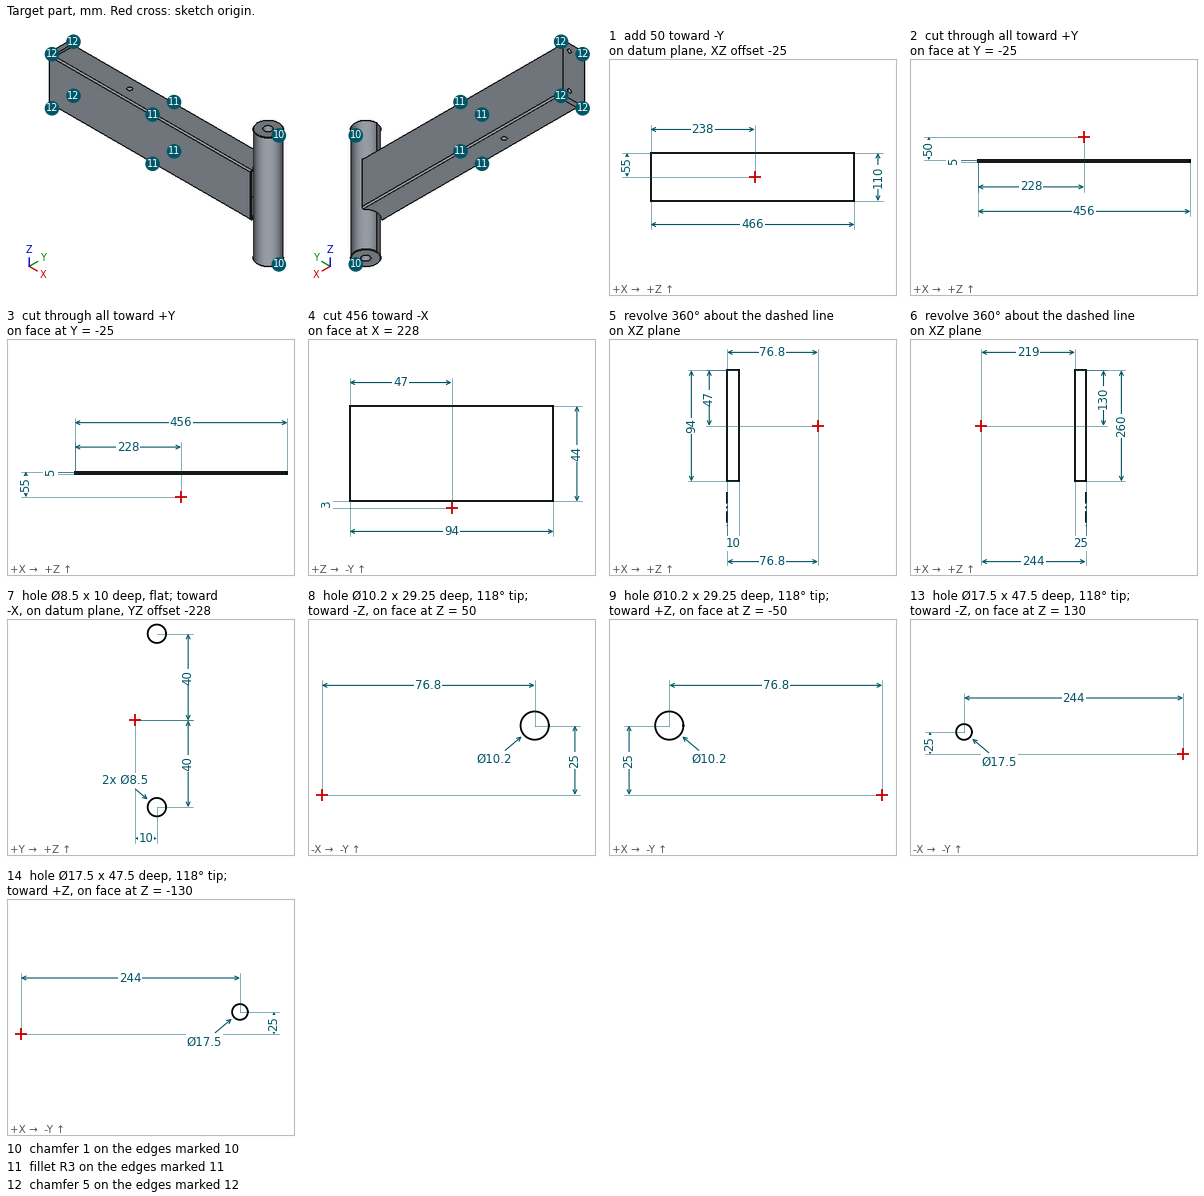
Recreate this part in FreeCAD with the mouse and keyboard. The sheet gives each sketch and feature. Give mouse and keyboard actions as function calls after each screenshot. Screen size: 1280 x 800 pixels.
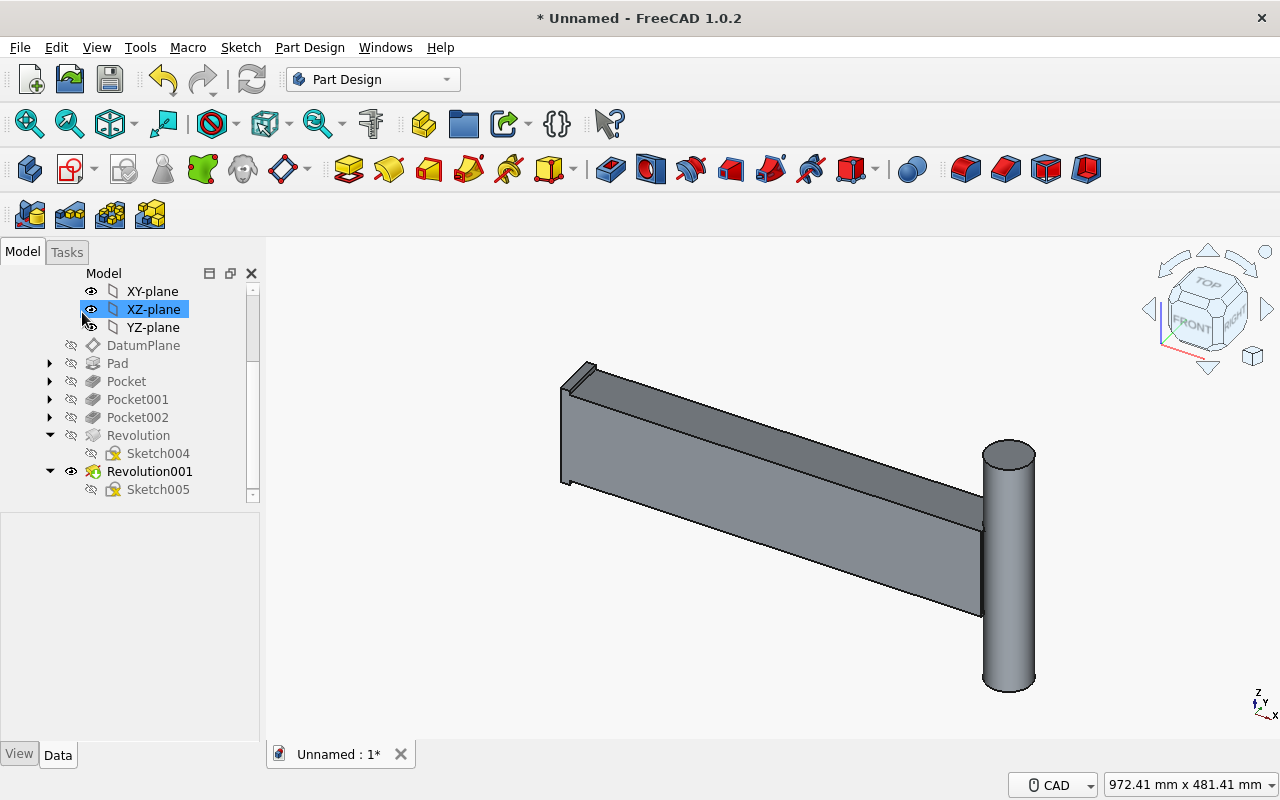
scroll(160, 395, down, 3)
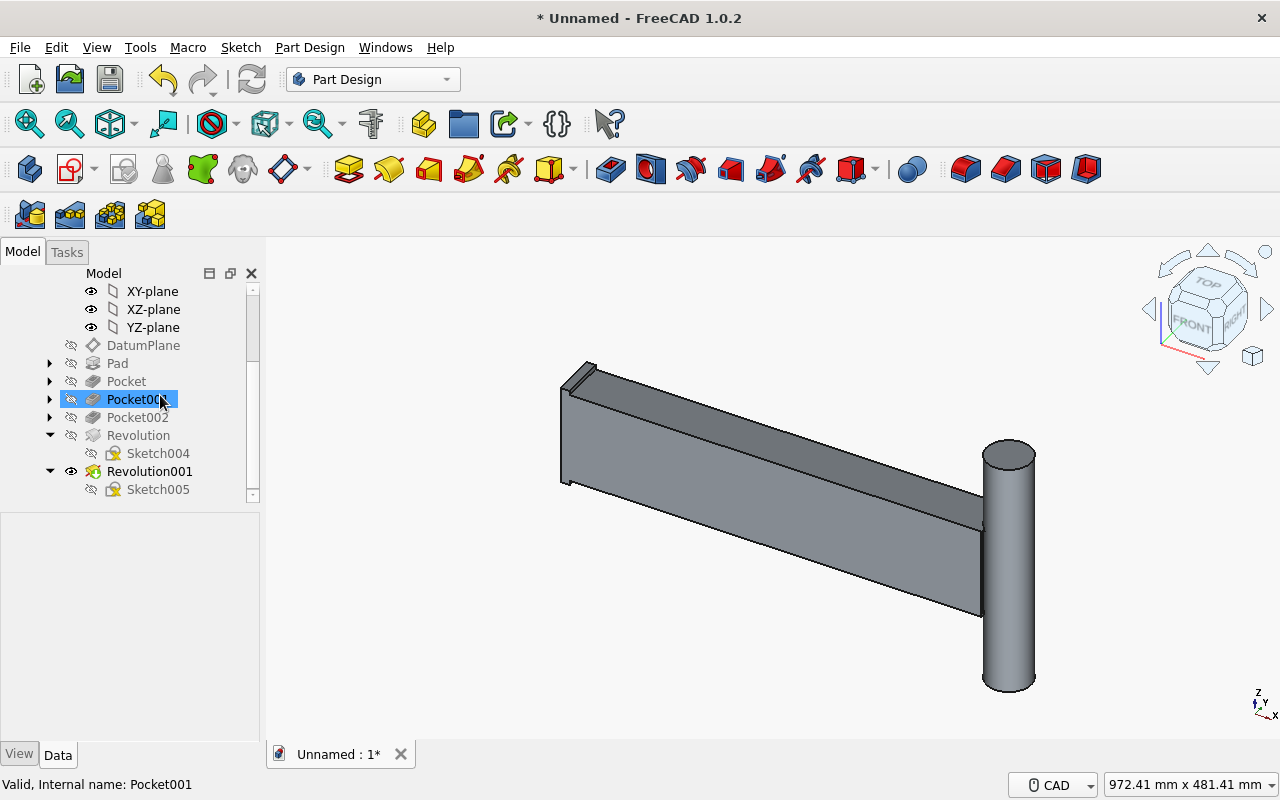
scroll(160, 395, up, 15)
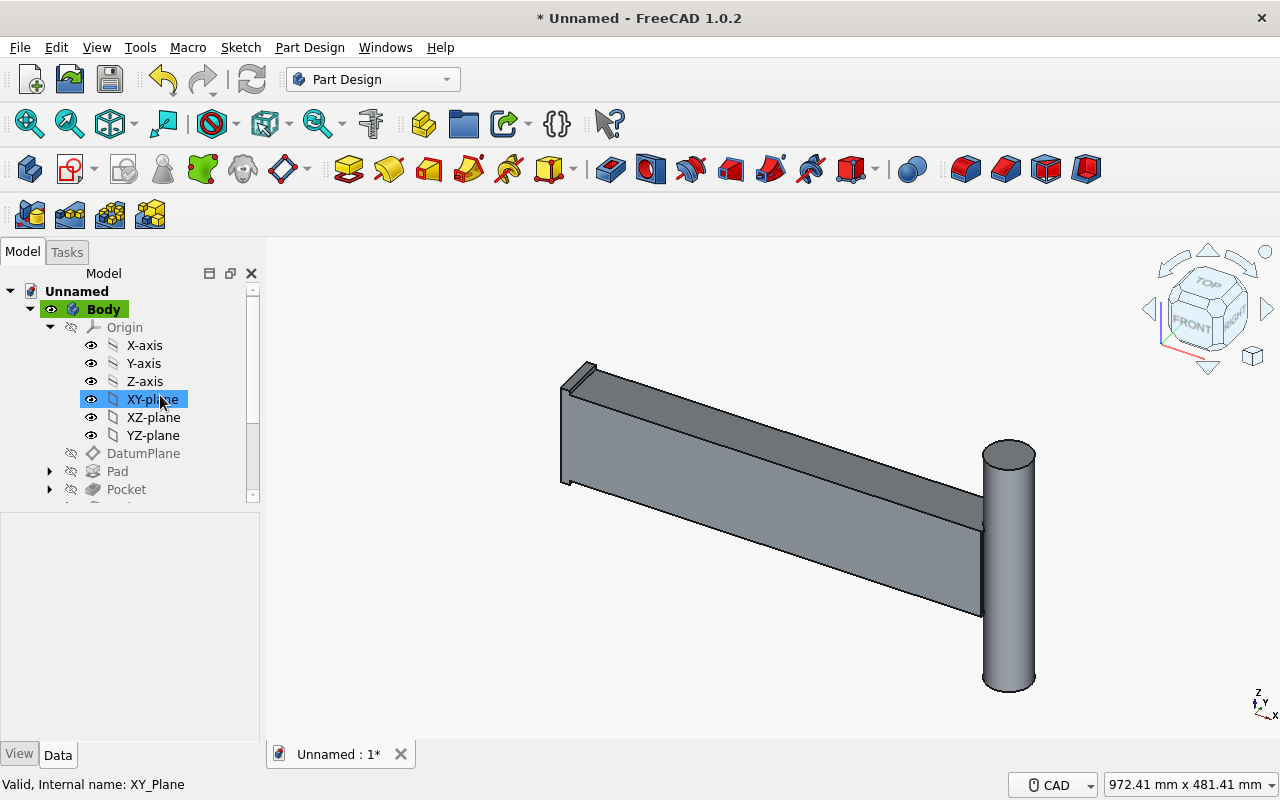
click(136, 435)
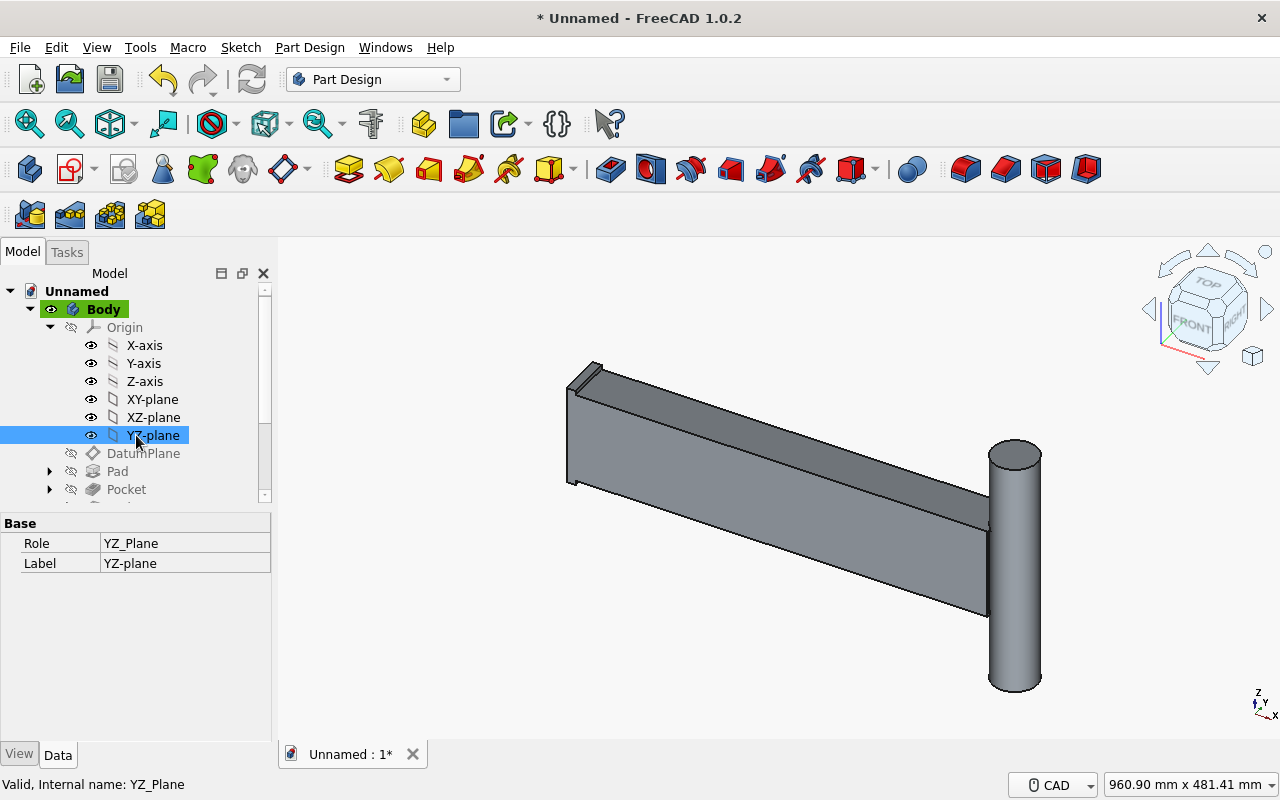
click(284, 170)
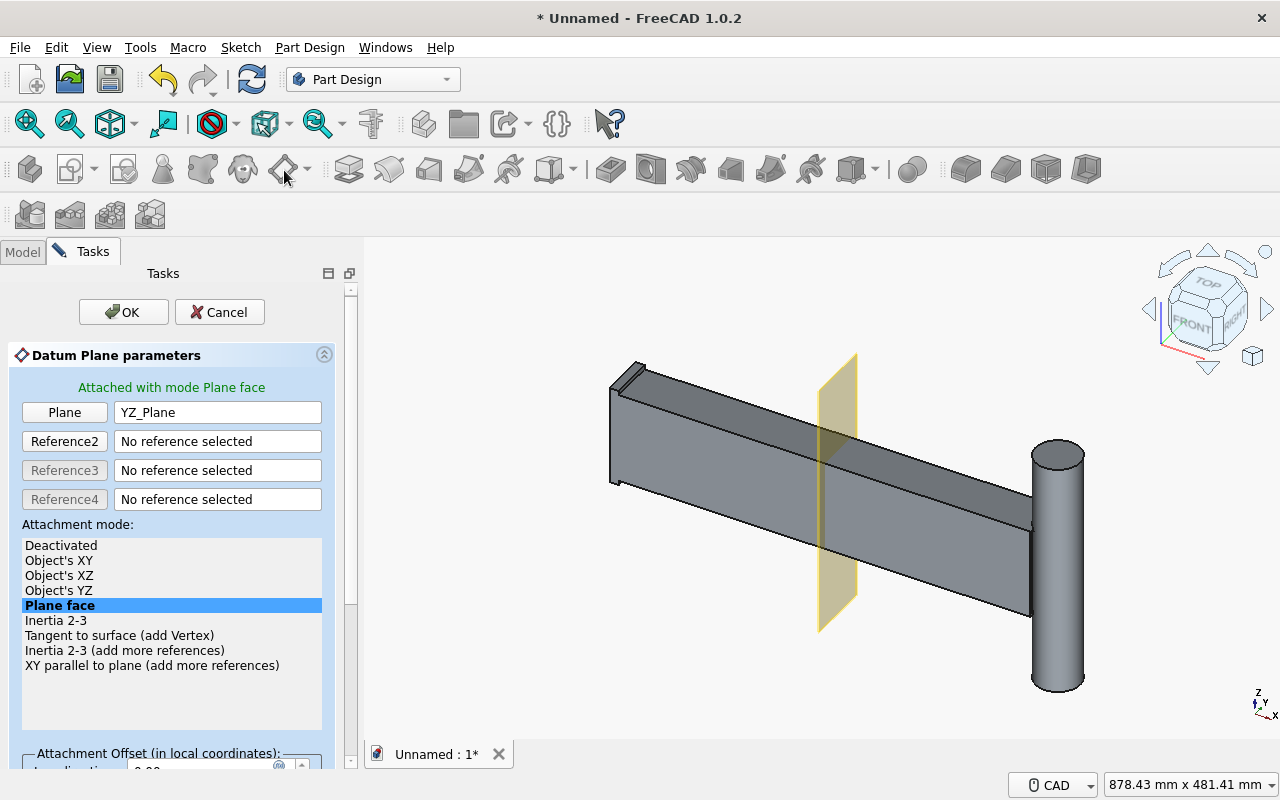
scroll(351, 526, down, 3)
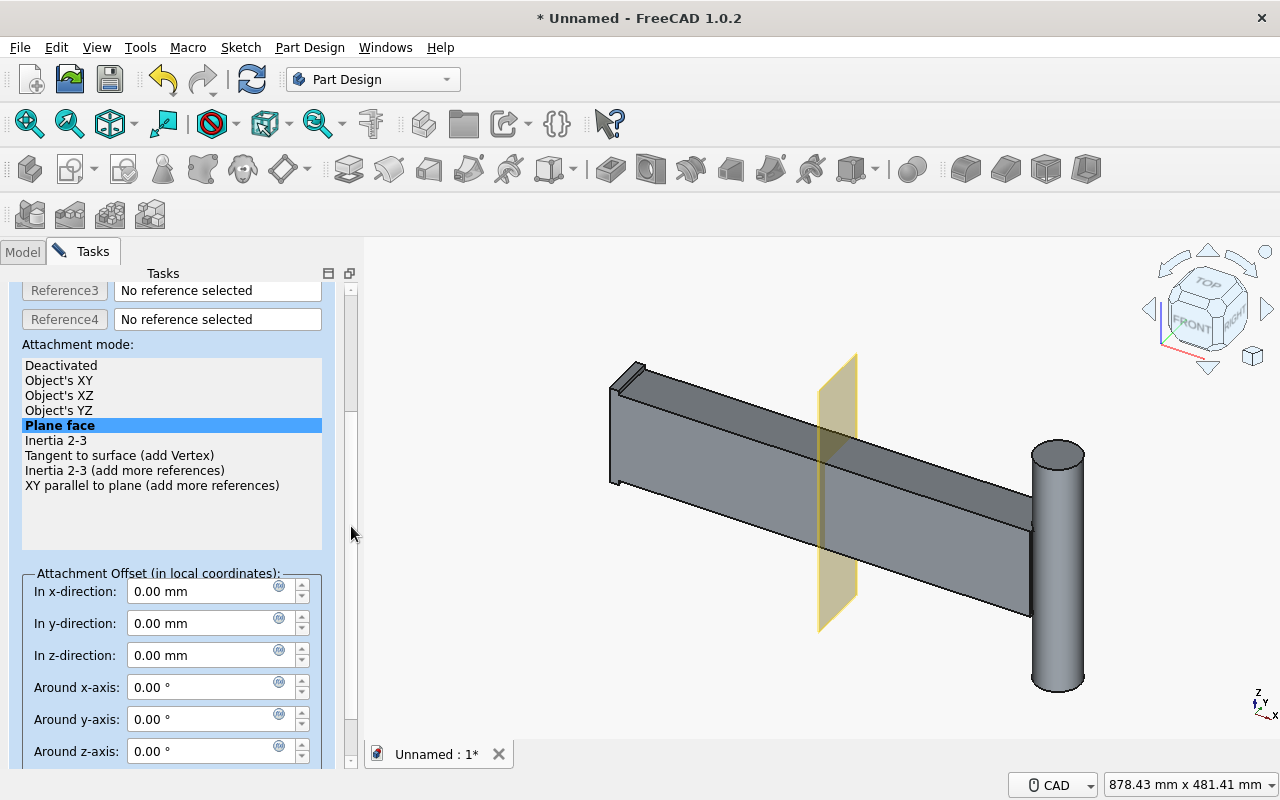
triple_click(210, 655)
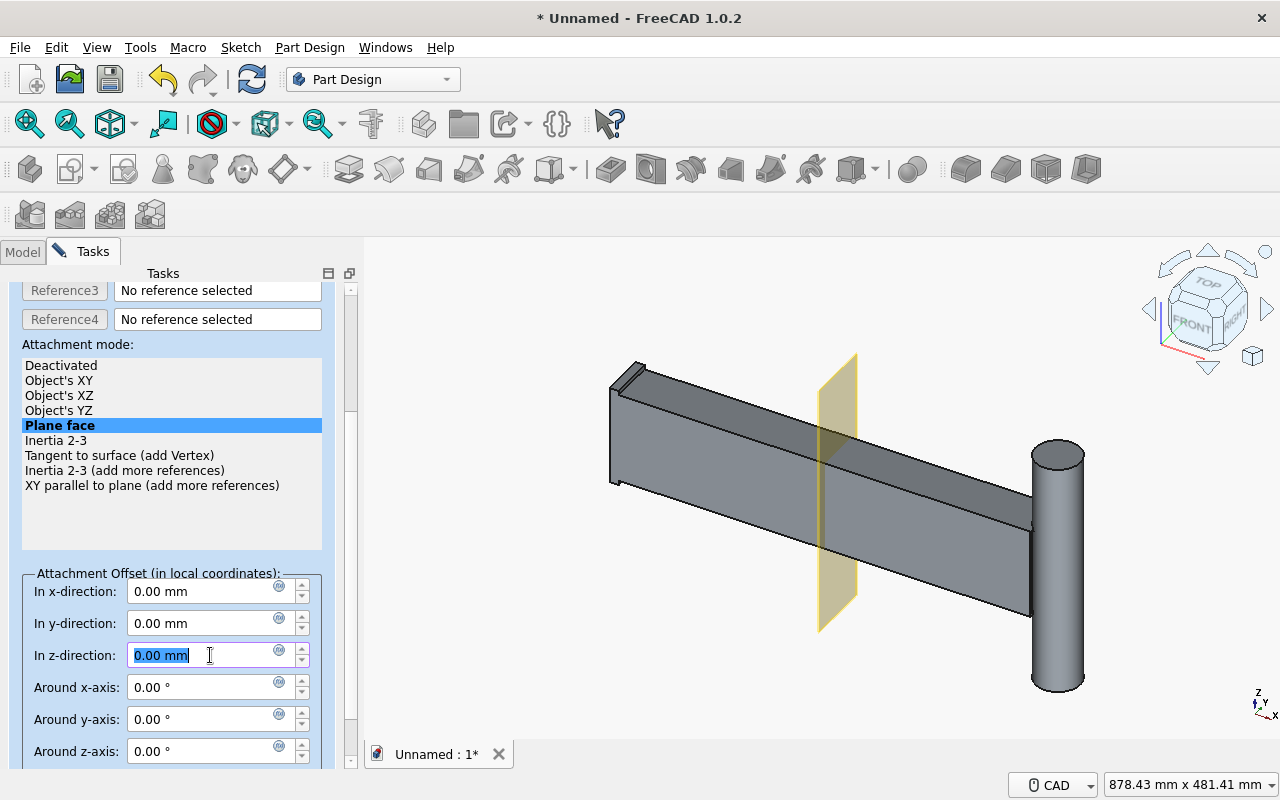
text(-228)
key(Tab)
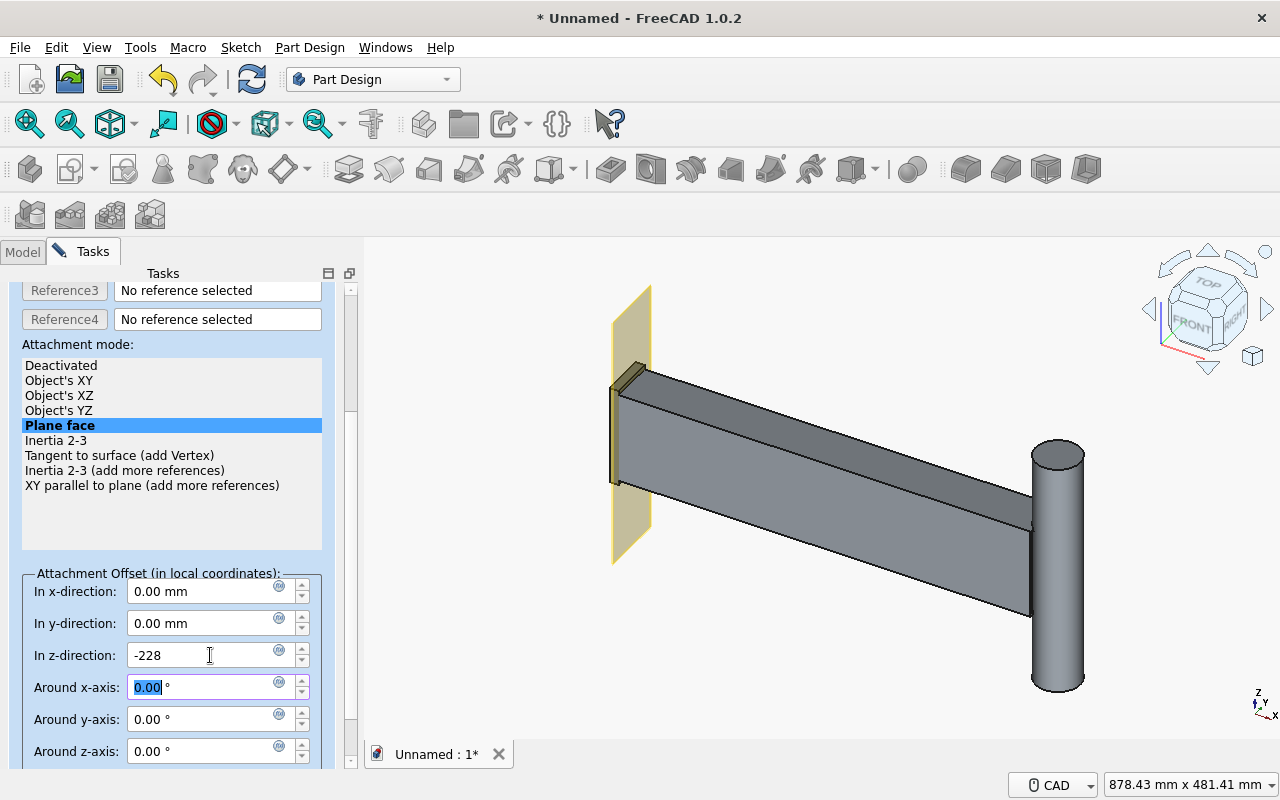
scroll(351, 526, up, 4)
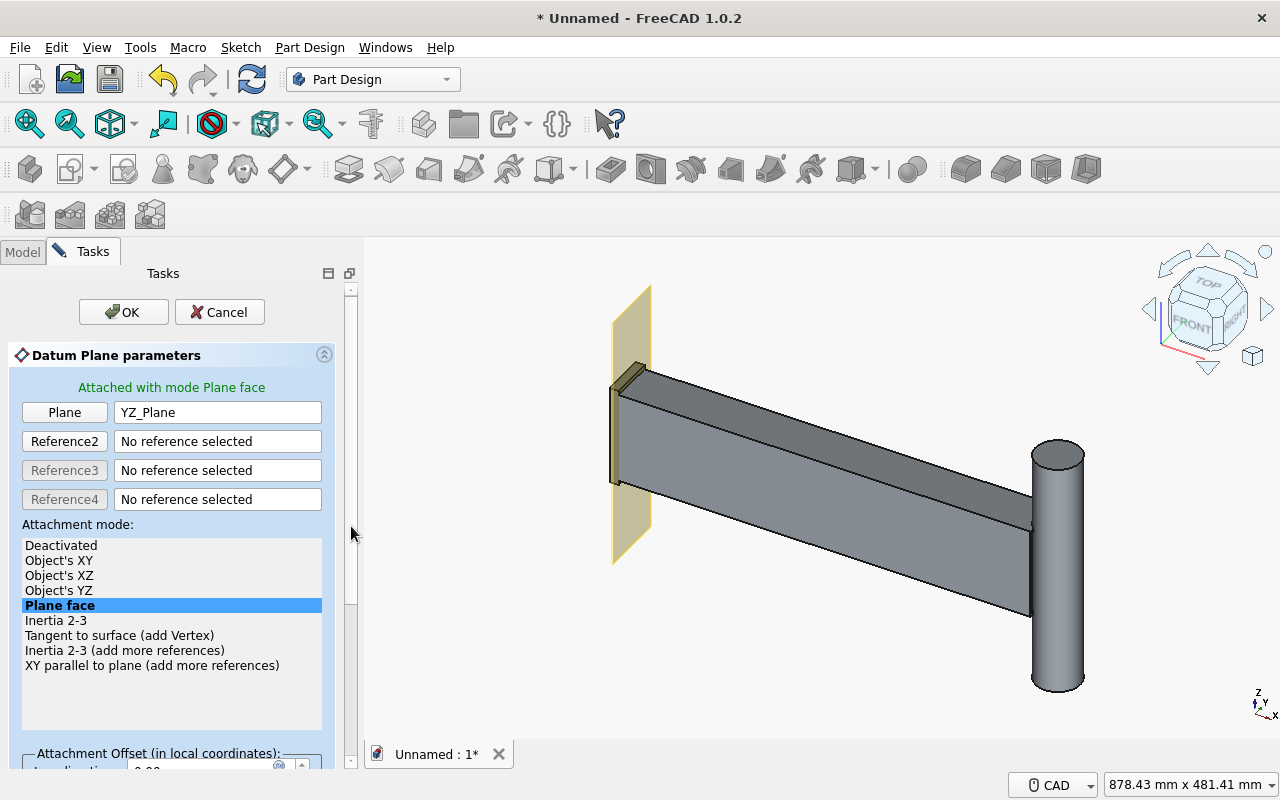
click(124, 312)